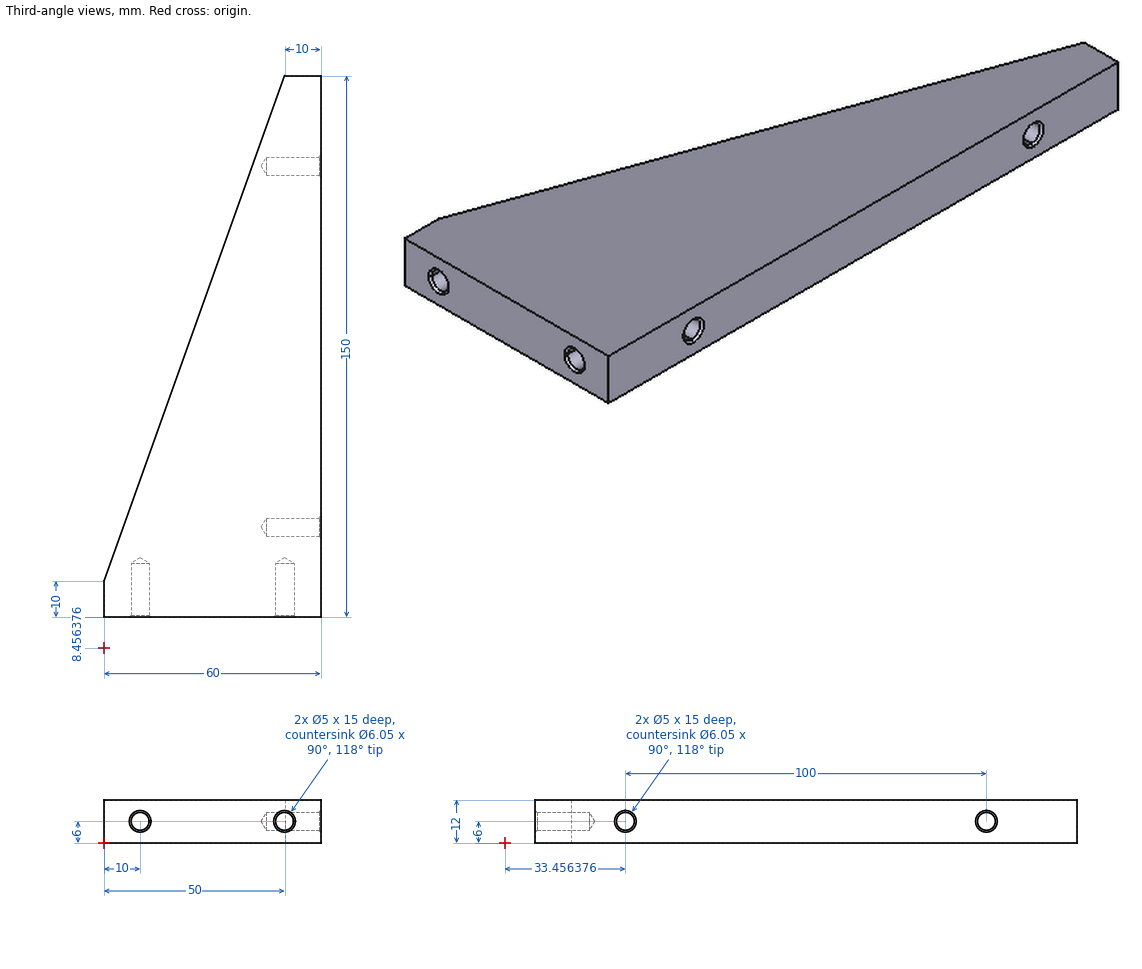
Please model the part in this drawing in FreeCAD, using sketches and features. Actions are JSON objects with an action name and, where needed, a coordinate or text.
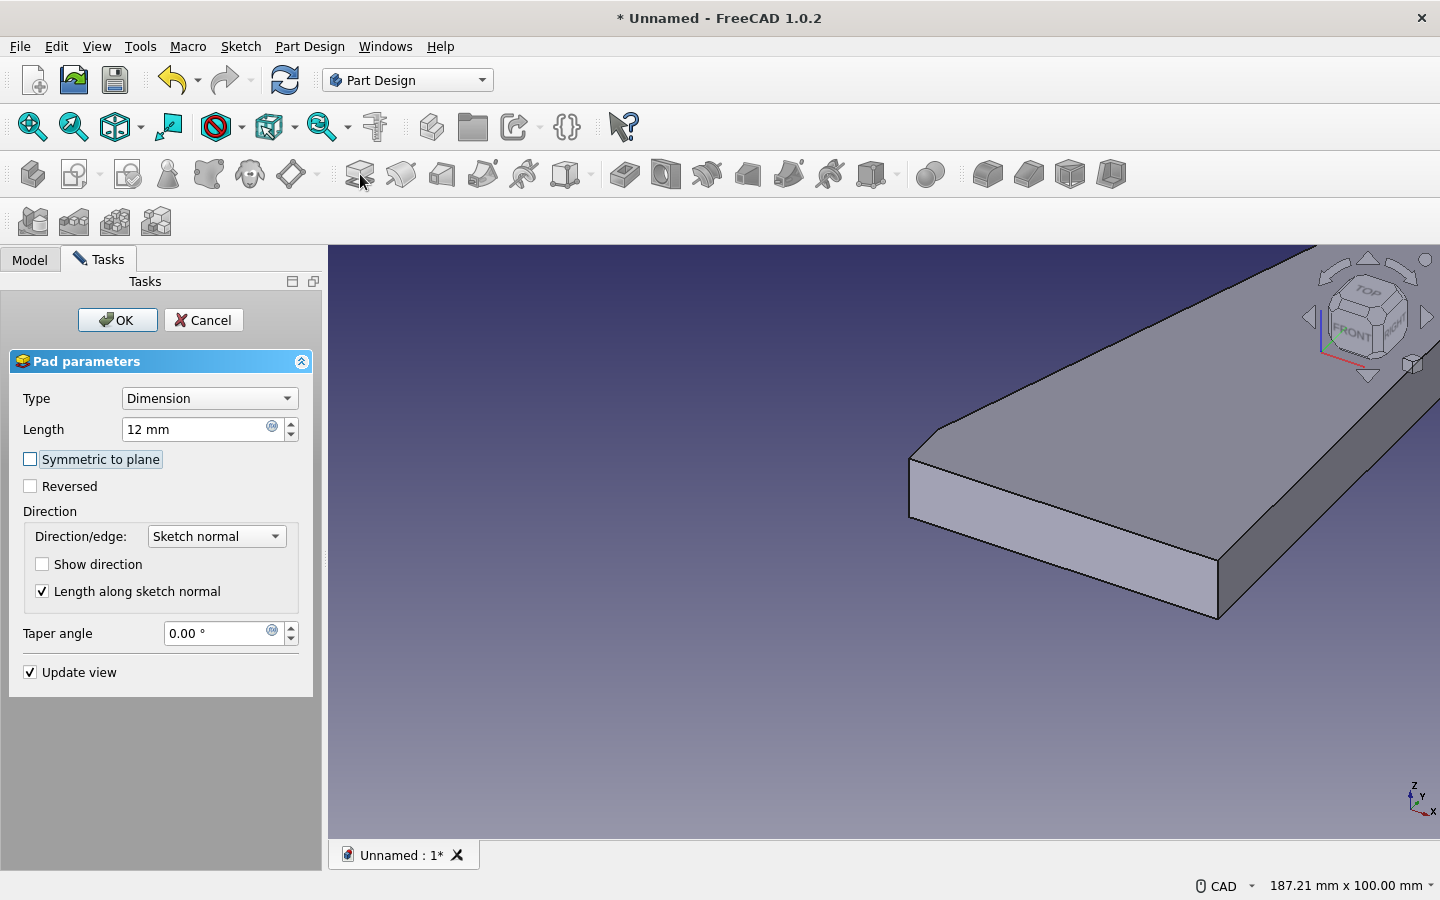
{"action": "left_click", "coordinate": [118, 320]}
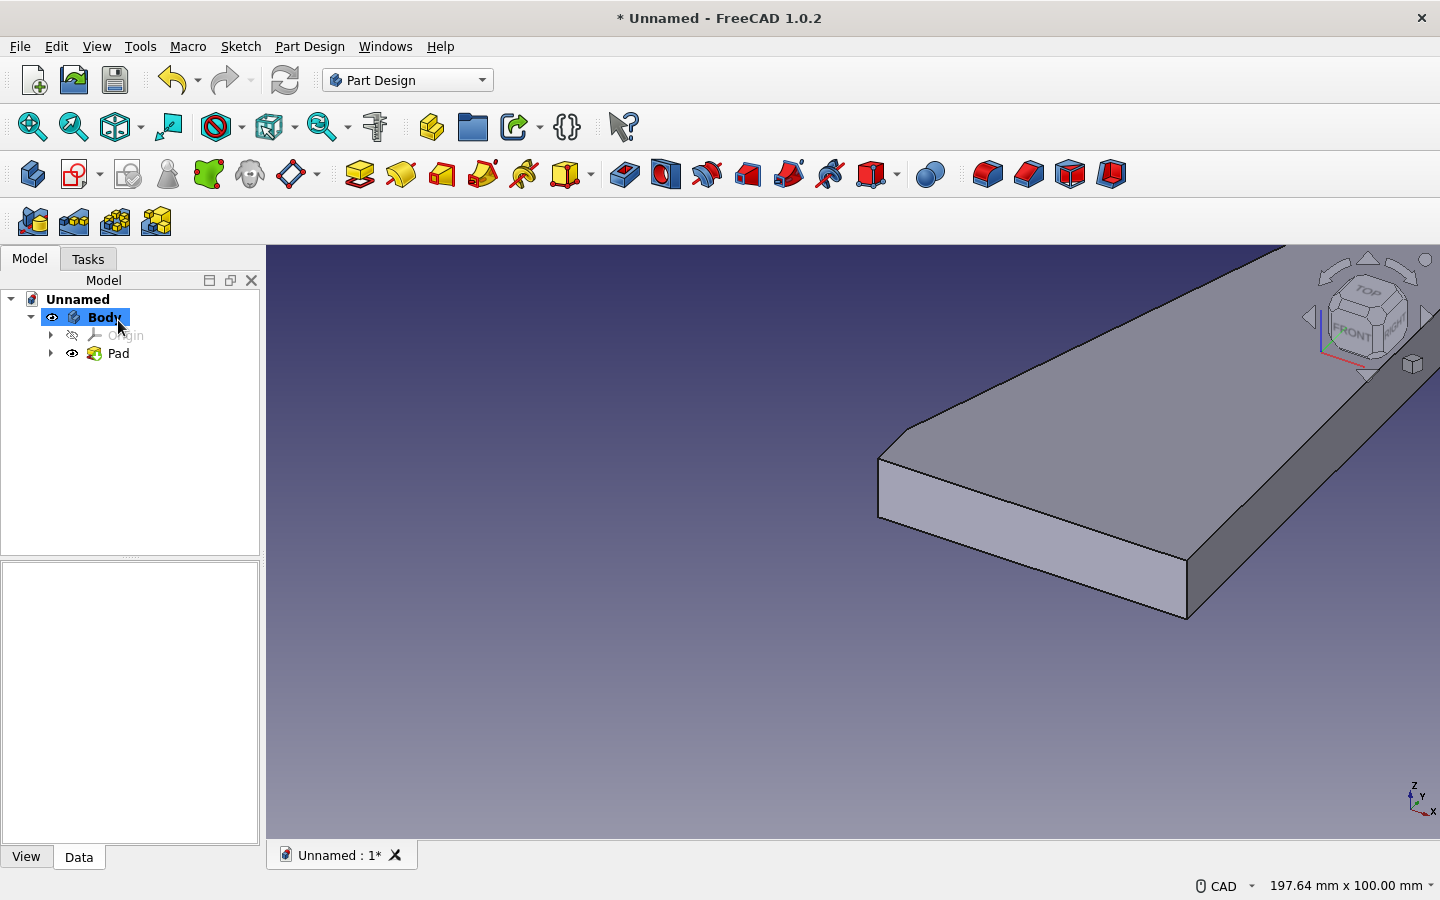
{"action": "left_click", "coordinate": [33, 128]}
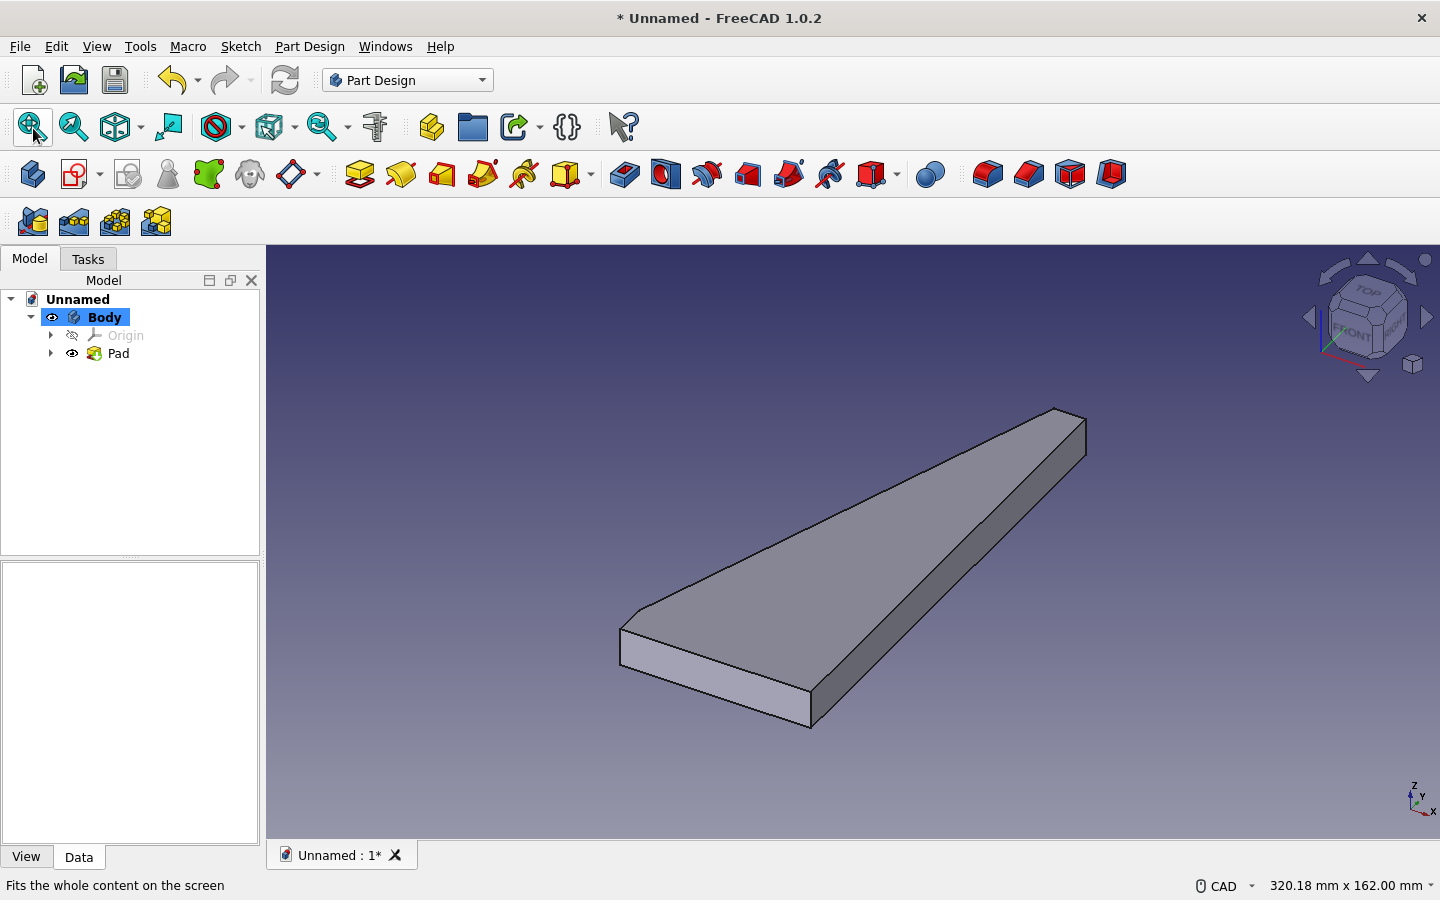
{"action": "left_click", "coordinate": [770, 696]}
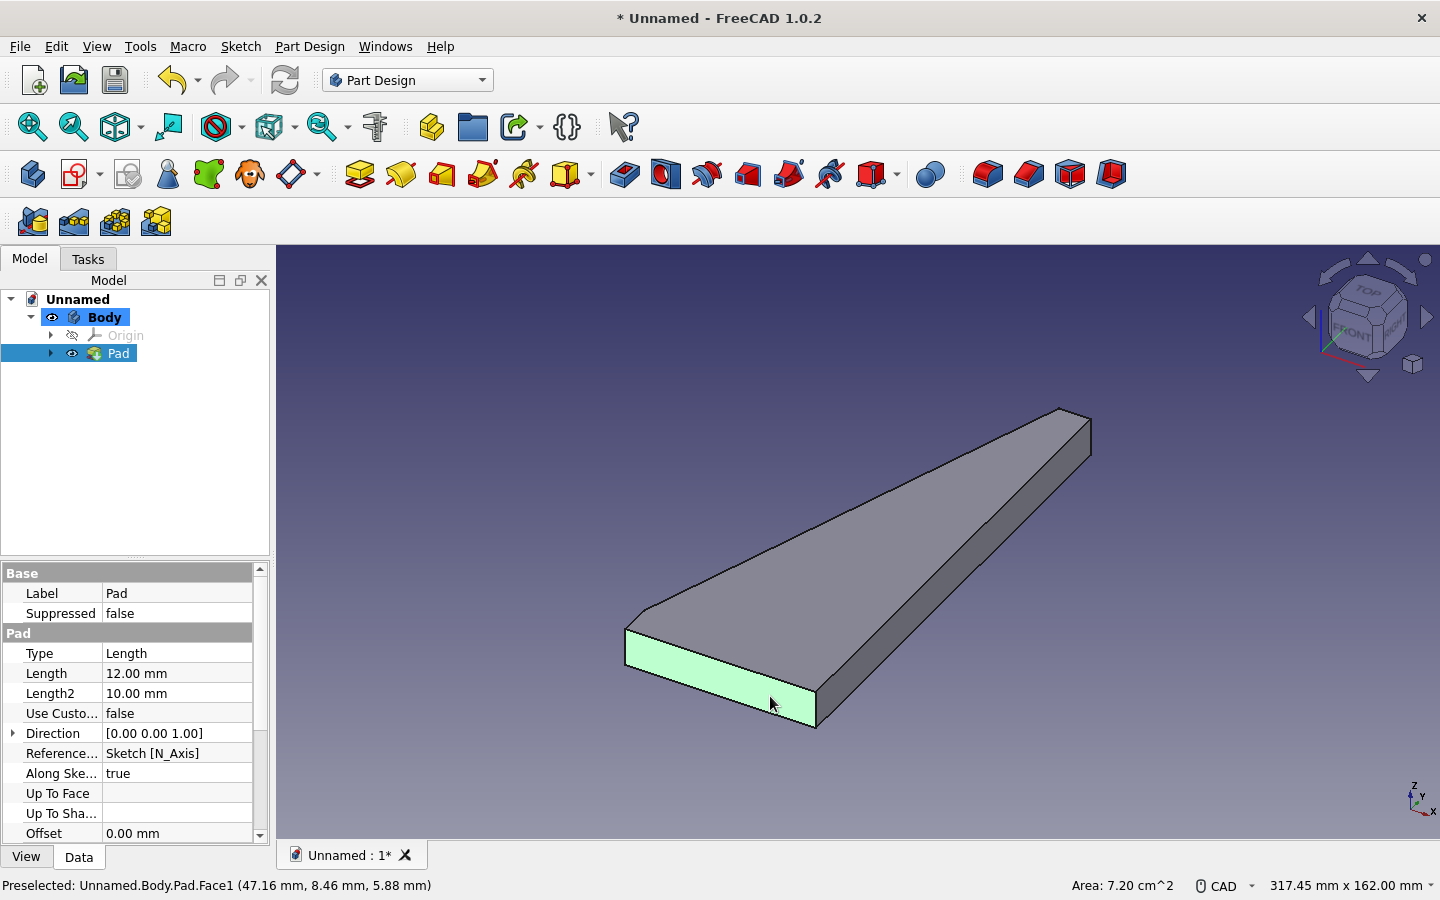
{"action": "left_click", "coordinate": [74, 174]}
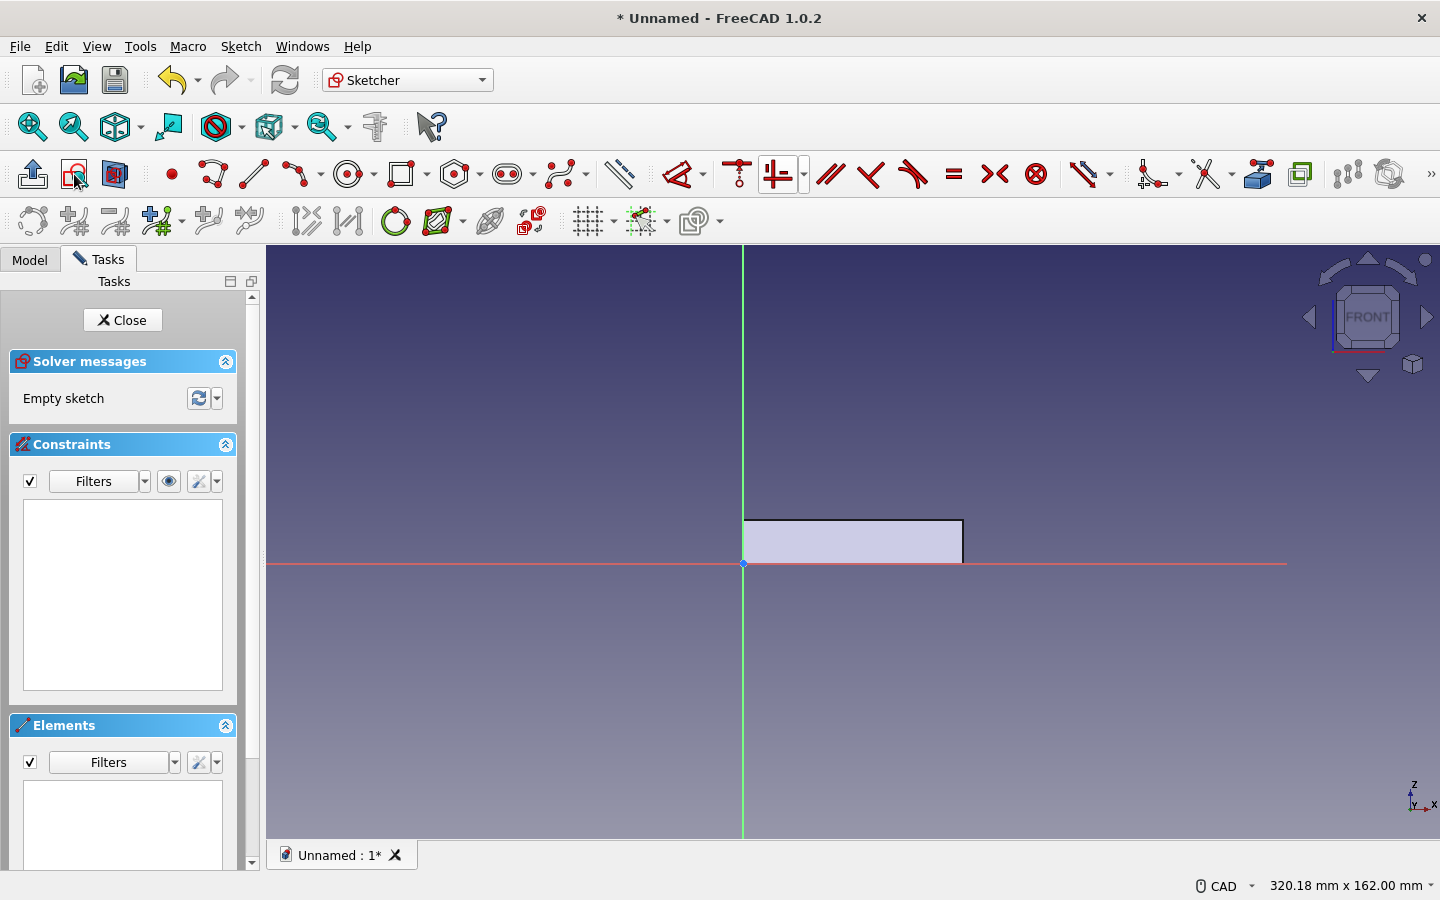
{"action": "scroll", "coordinate": [863, 551], "scroll_direction": "up", "scroll_amount": 6}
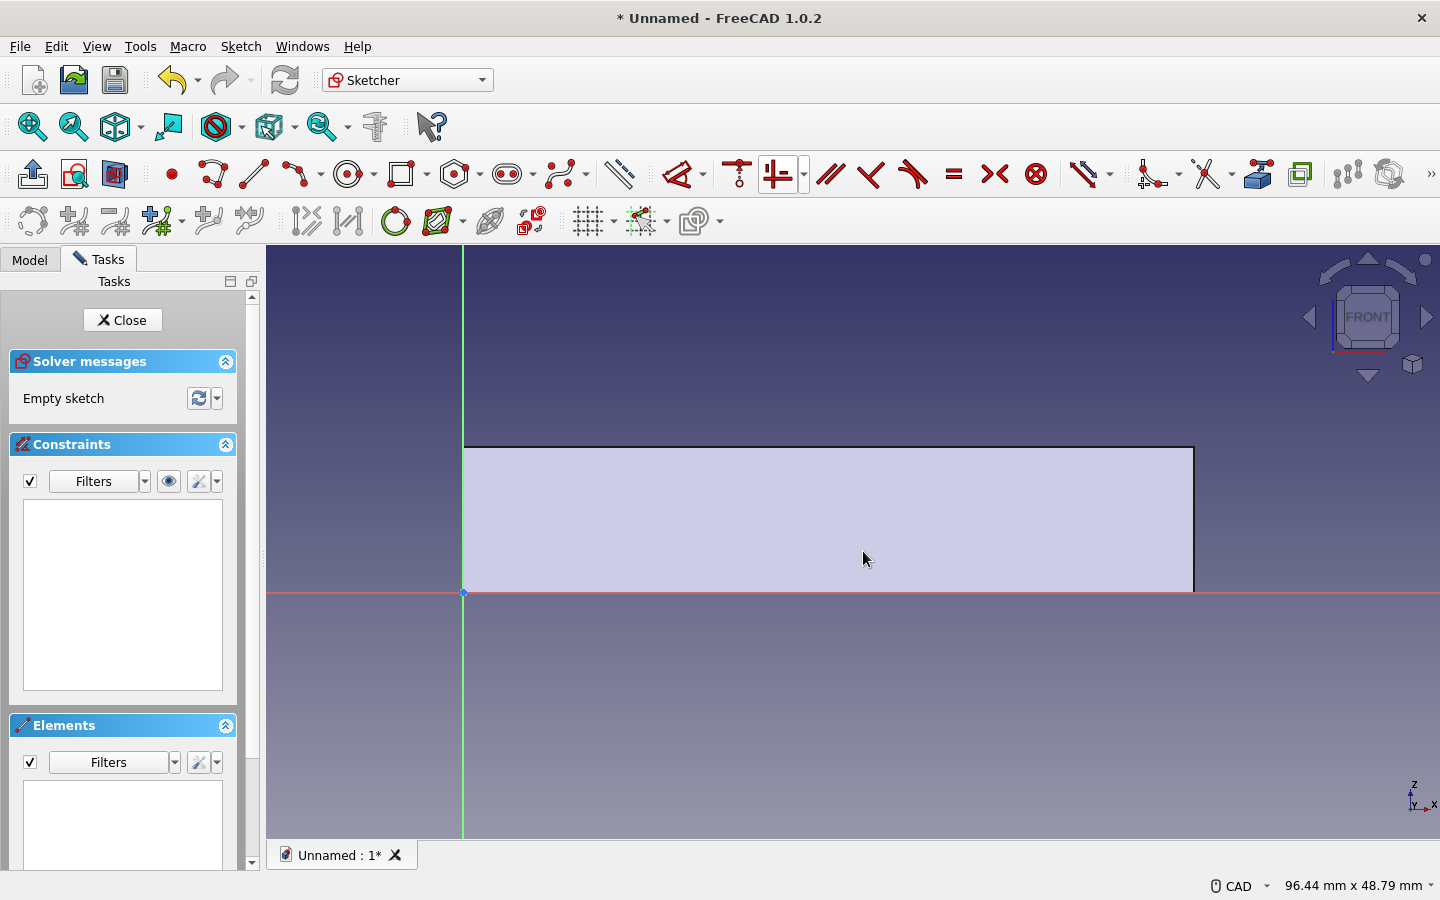
{"action": "left_click", "coordinate": [348, 174]}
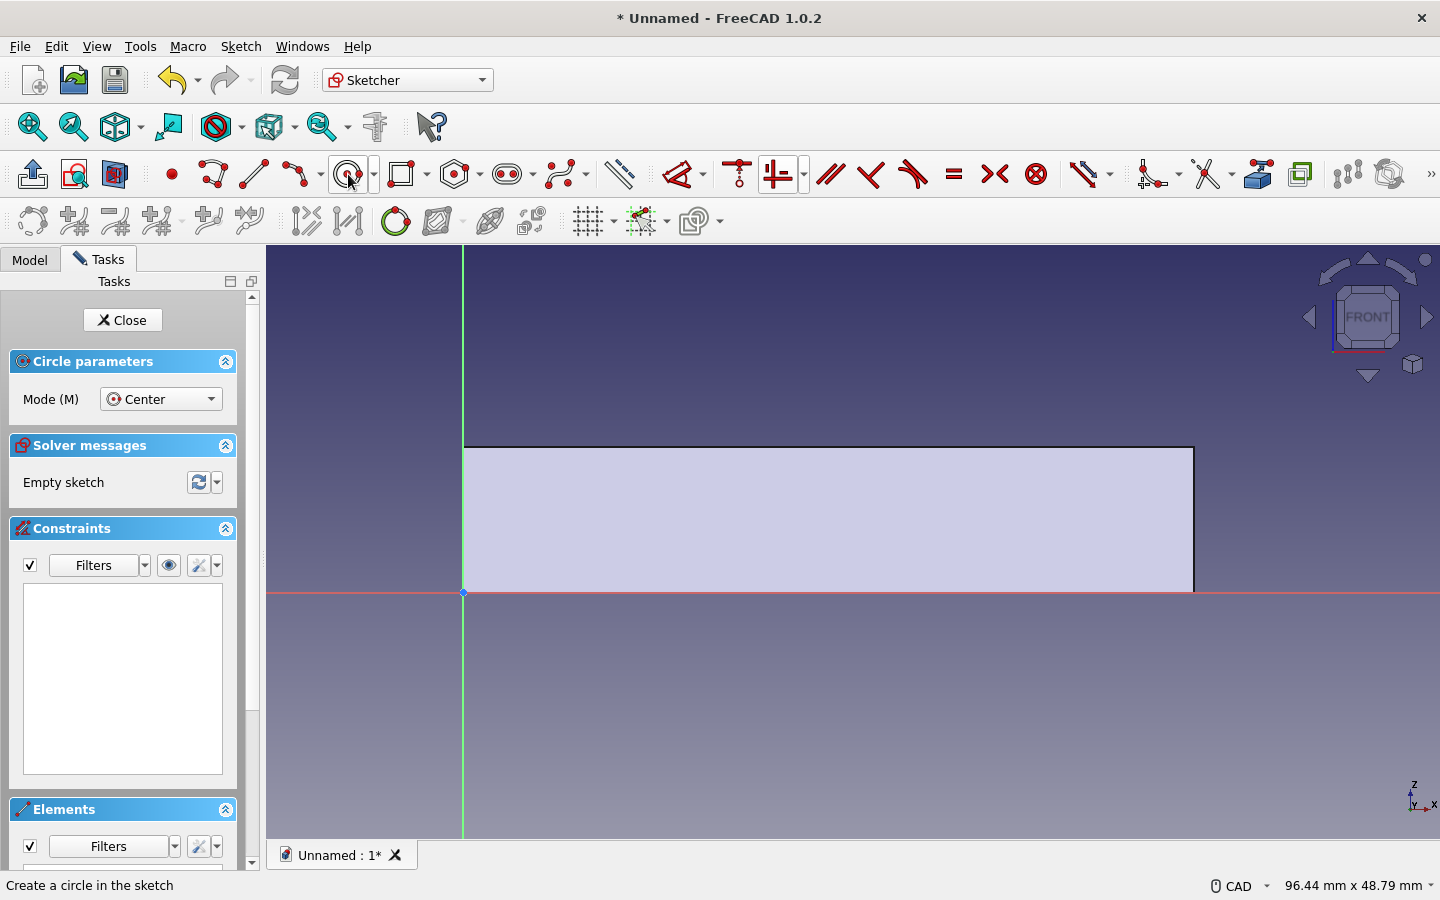
{"action": "left_click", "coordinate": [1072, 520]}
{"action": "mouse_move", "coordinate": [1094, 498]}